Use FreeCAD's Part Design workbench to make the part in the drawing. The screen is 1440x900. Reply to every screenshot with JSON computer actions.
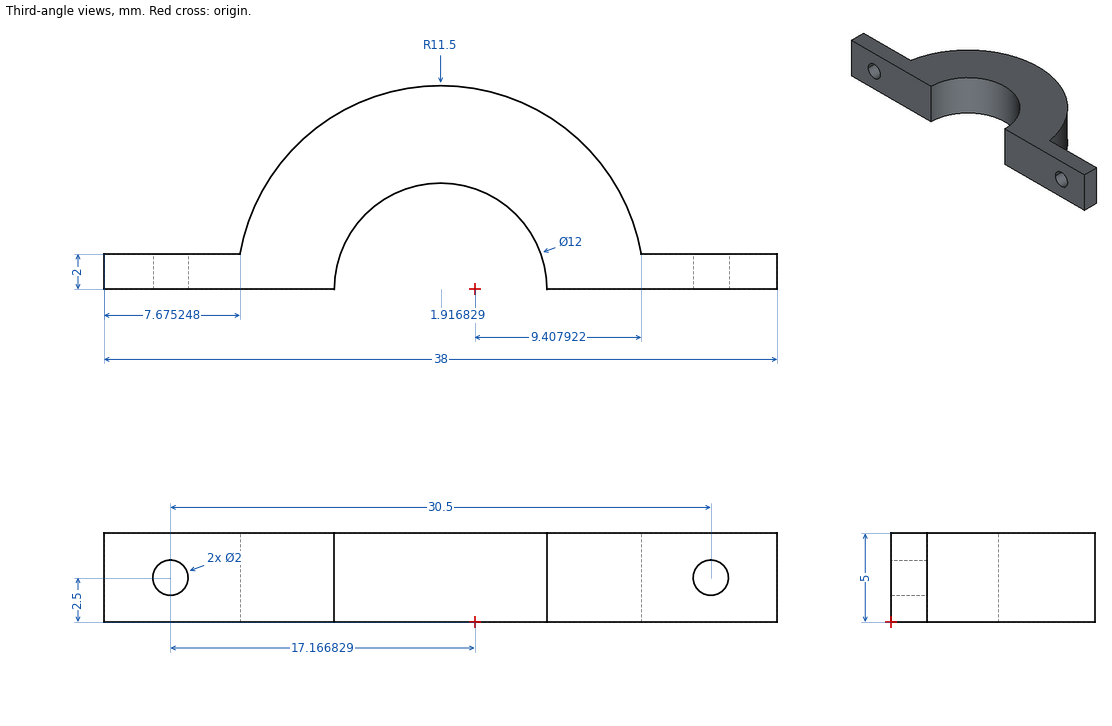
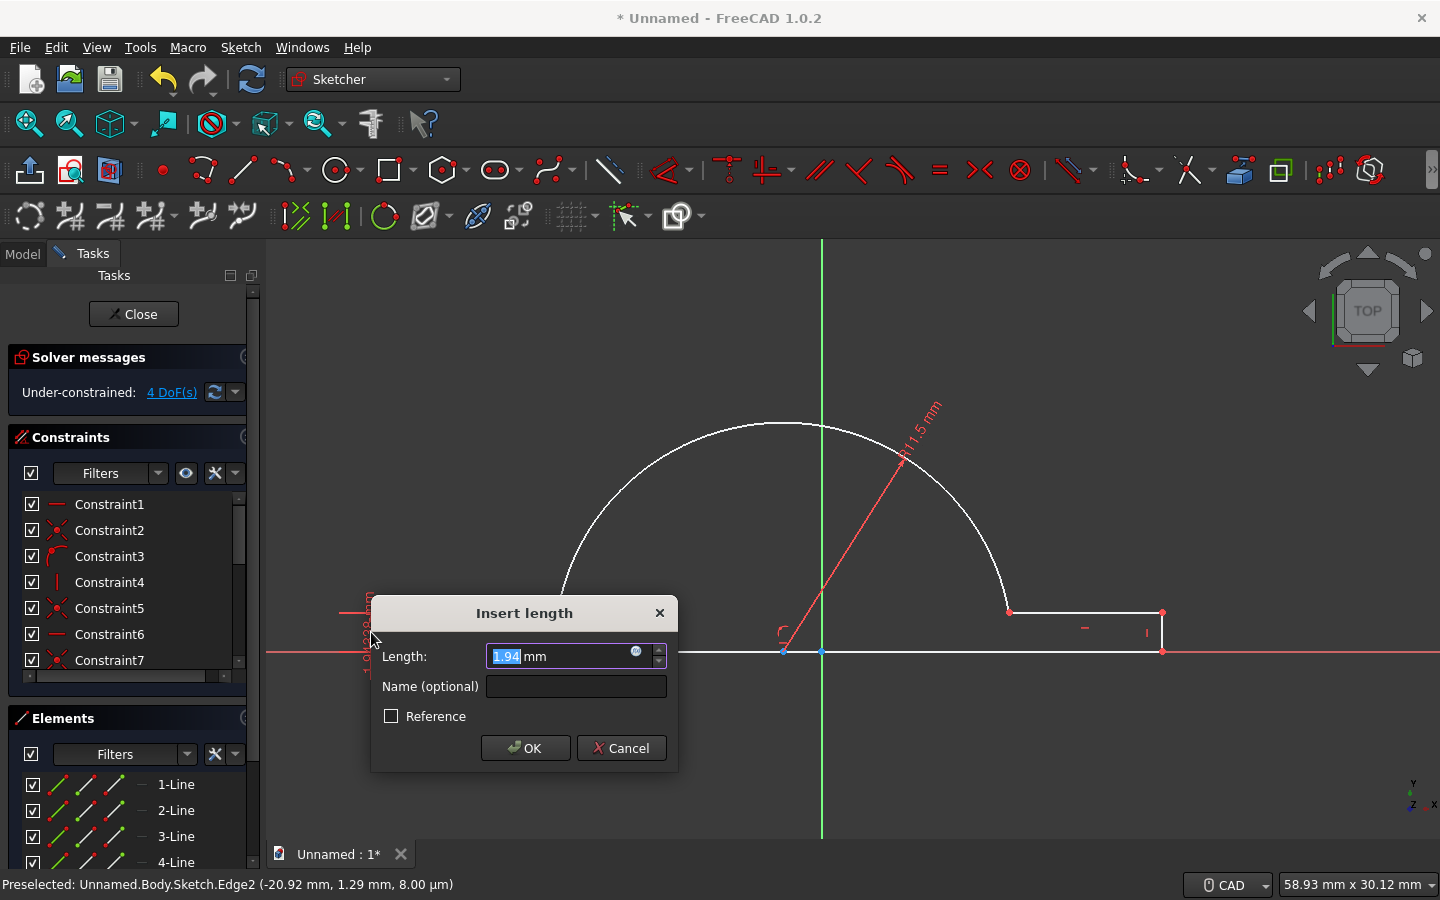
{"action": "type", "text": "2"}
{"action": "key", "text": "Return"}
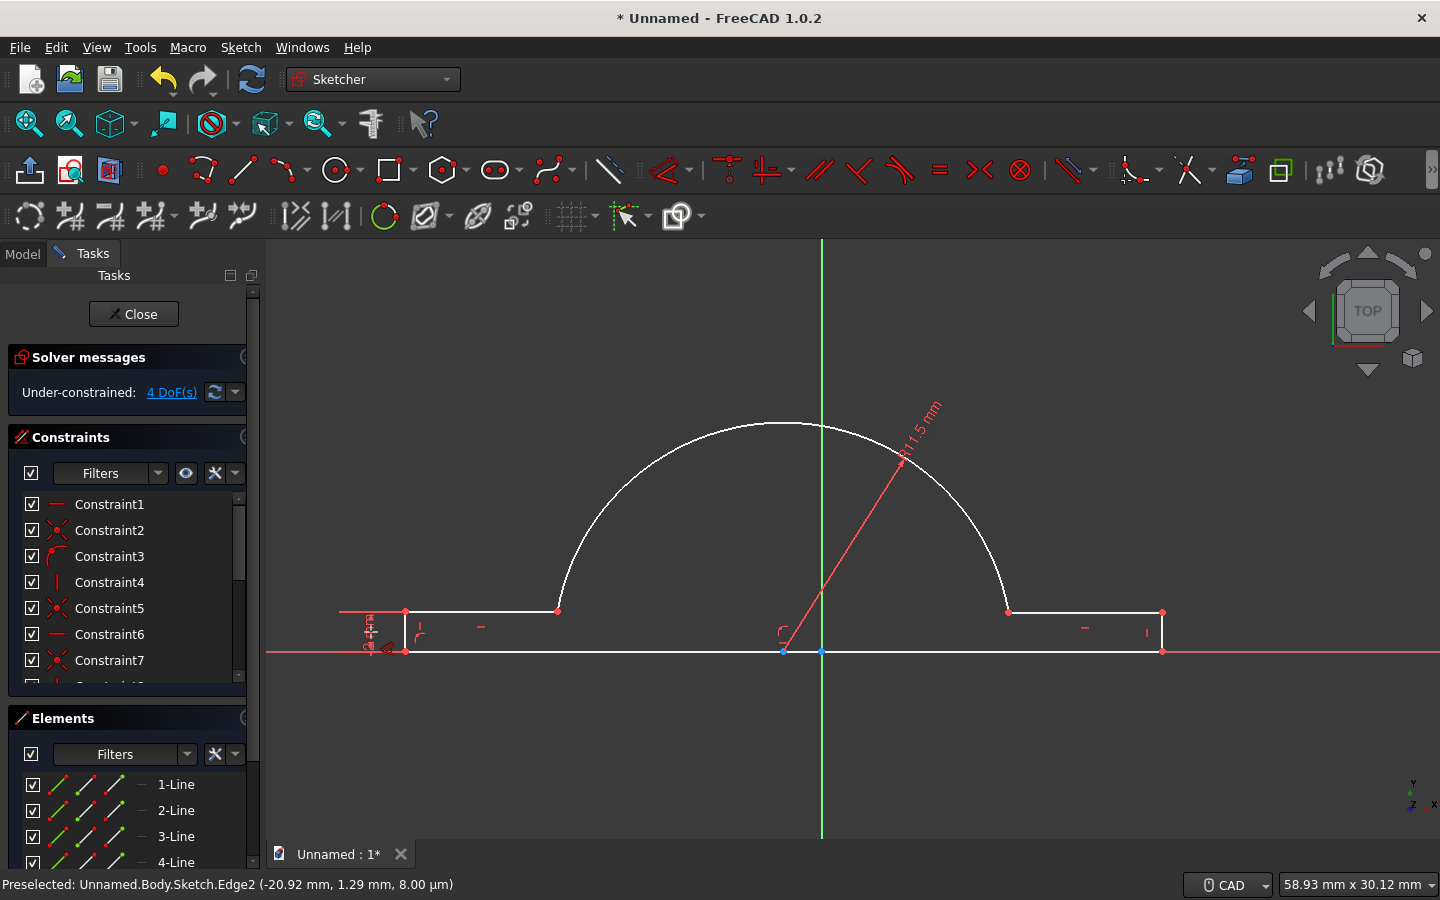
{"action": "left_click", "coordinate": [1162, 640]}
{"action": "left_click", "coordinate": [1196, 632]}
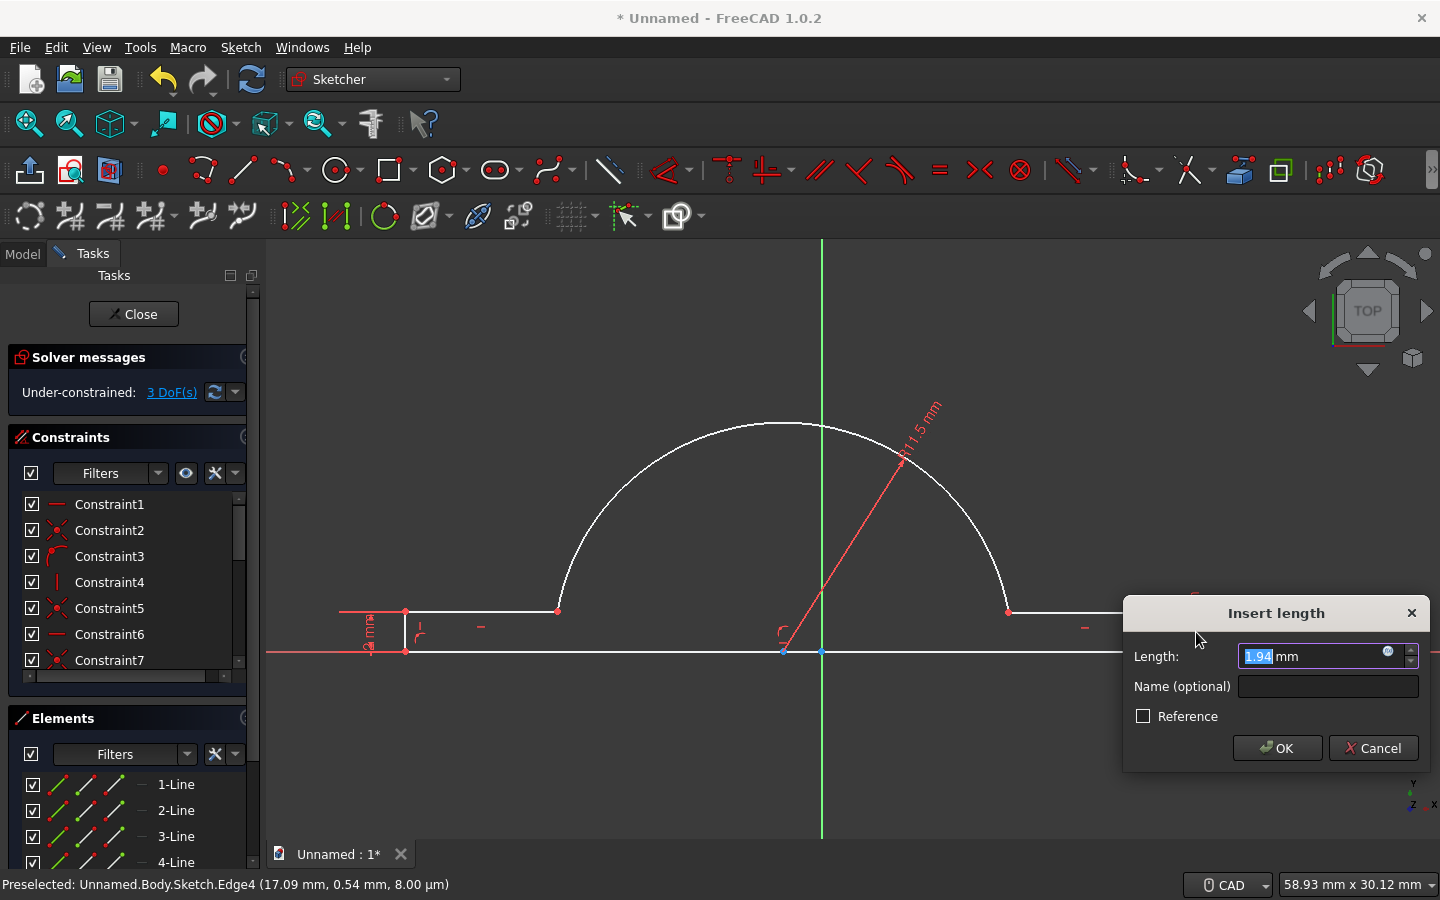
{"action": "type", "text": "2"}
{"action": "key", "text": "Return"}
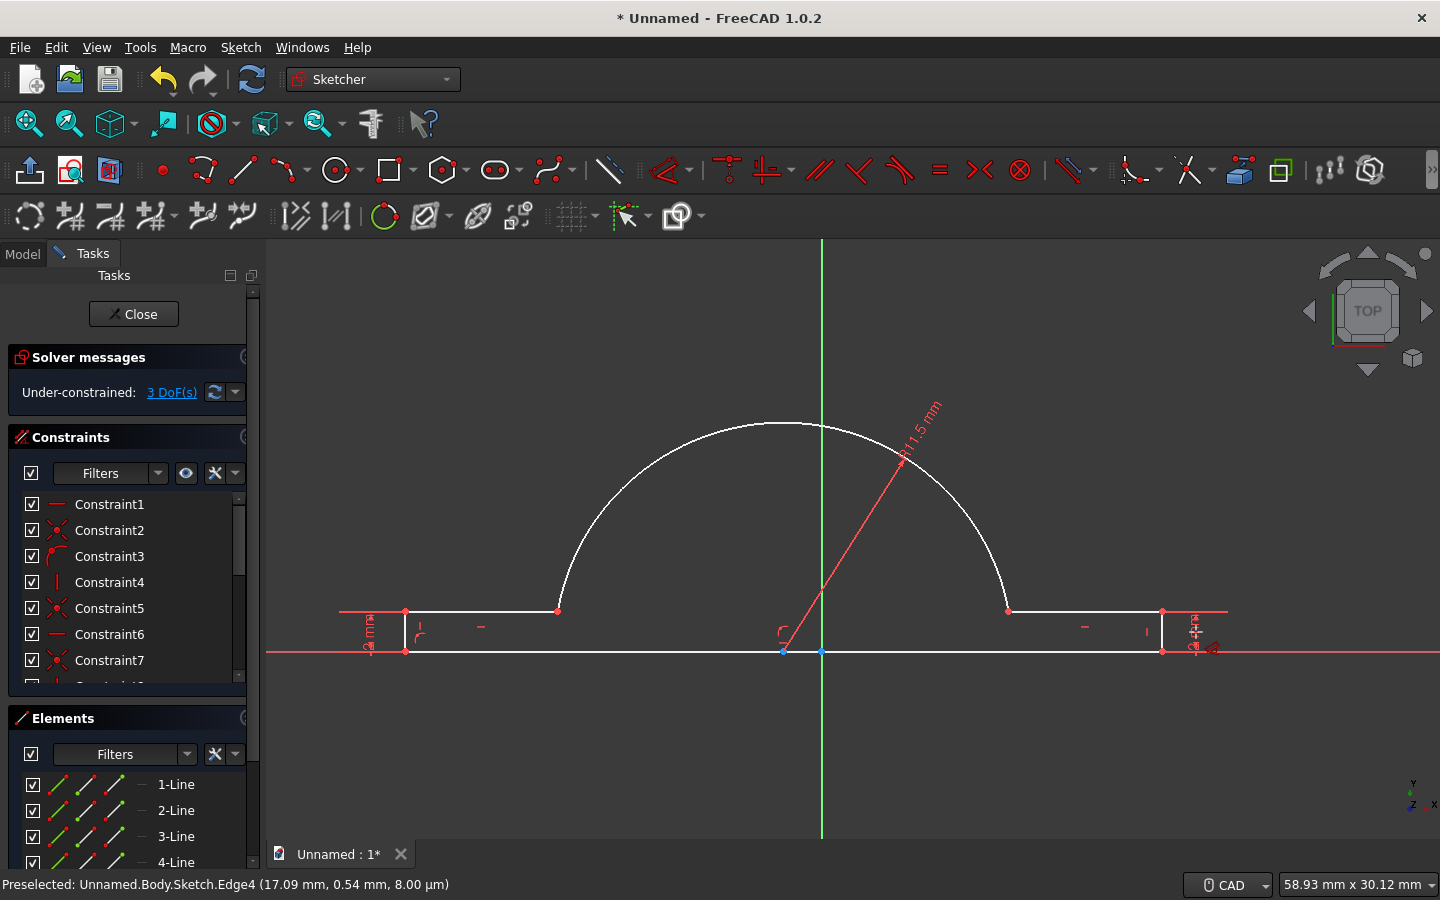
{"action": "left_click", "coordinate": [632, 652]}
{"action": "left_click", "coordinate": [783, 686]}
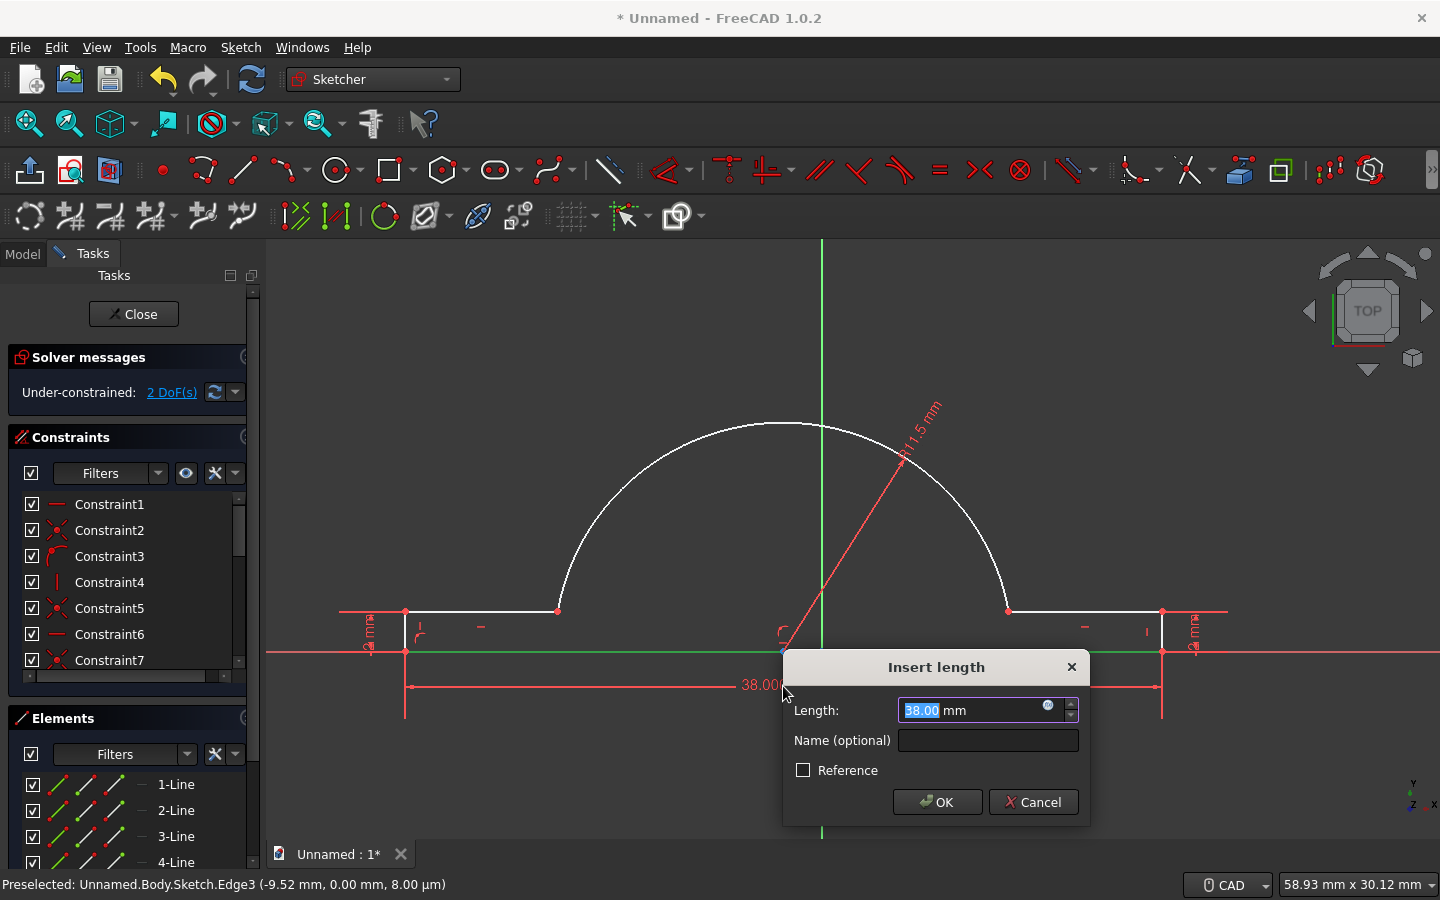
{"action": "type", "text": "38"}
{"action": "key", "text": "Return"}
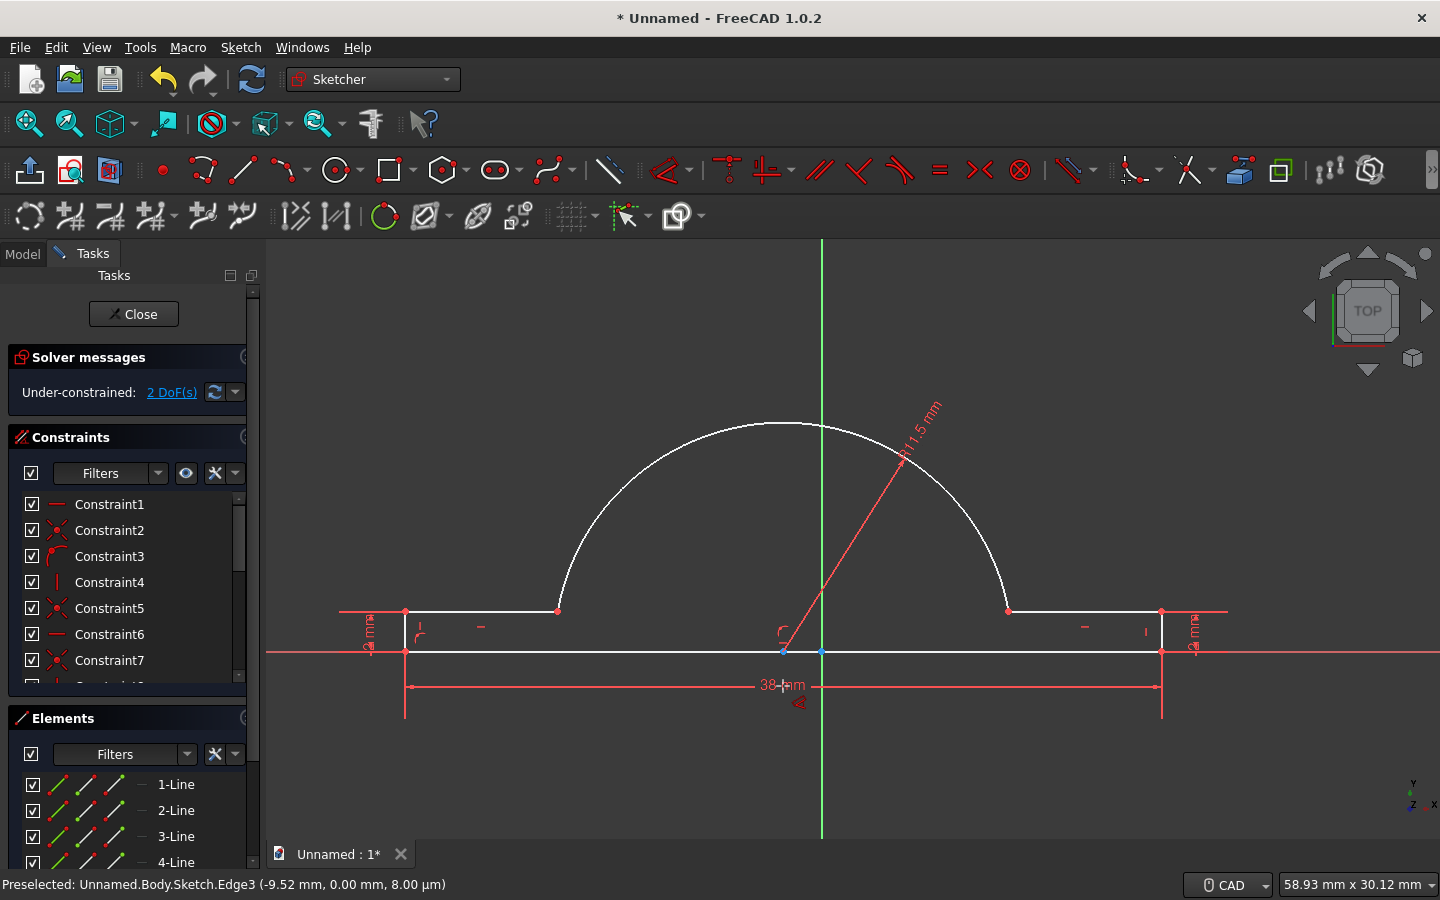
{"action": "left_click", "coordinate": [512, 612]}
{"action": "left_click", "coordinate": [481, 578]}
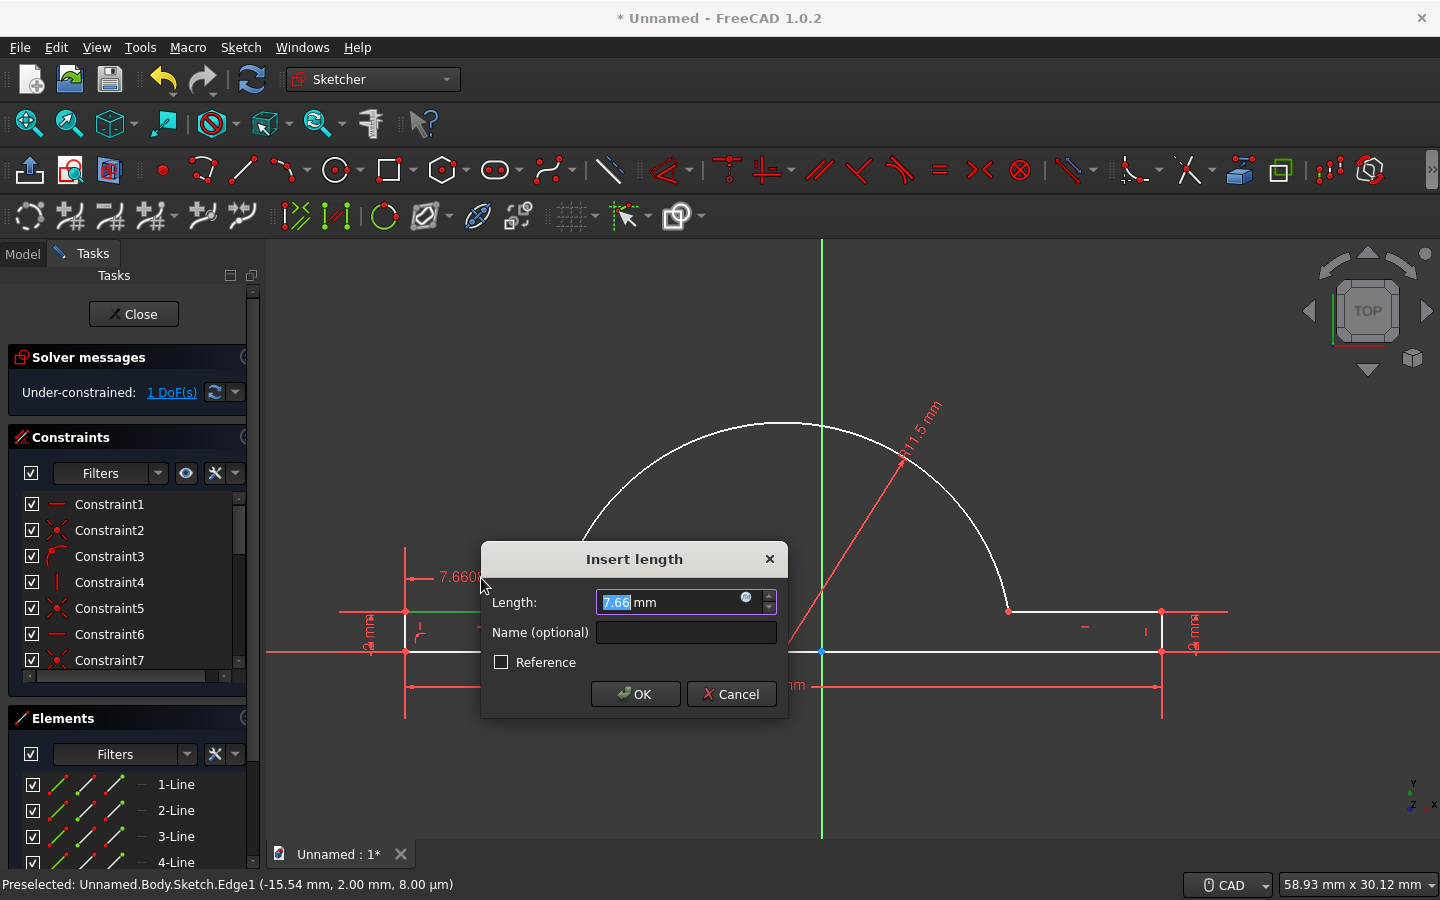
{"action": "type", "text": "7.675248"}
{"action": "key", "text": "Return"}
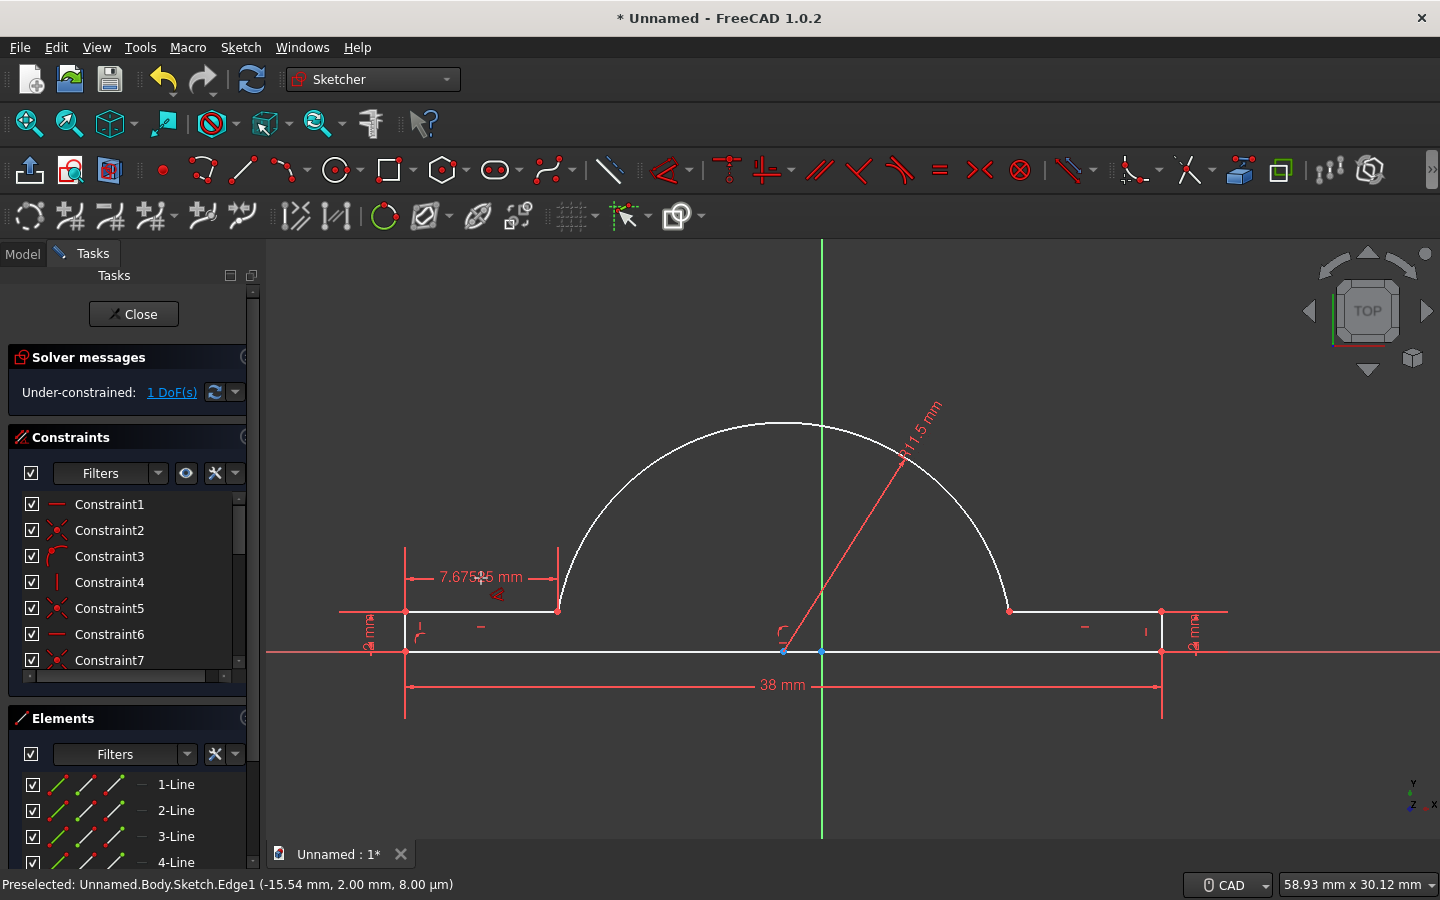
{"action": "left_click", "coordinate": [1009, 612]}
{"action": "left_click", "coordinate": [915, 686]}